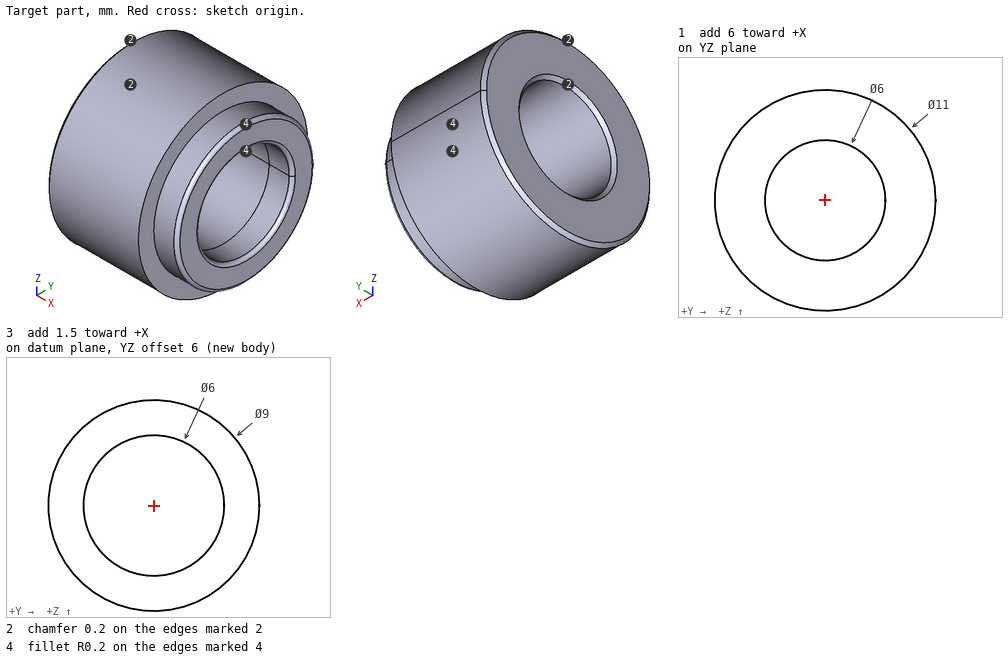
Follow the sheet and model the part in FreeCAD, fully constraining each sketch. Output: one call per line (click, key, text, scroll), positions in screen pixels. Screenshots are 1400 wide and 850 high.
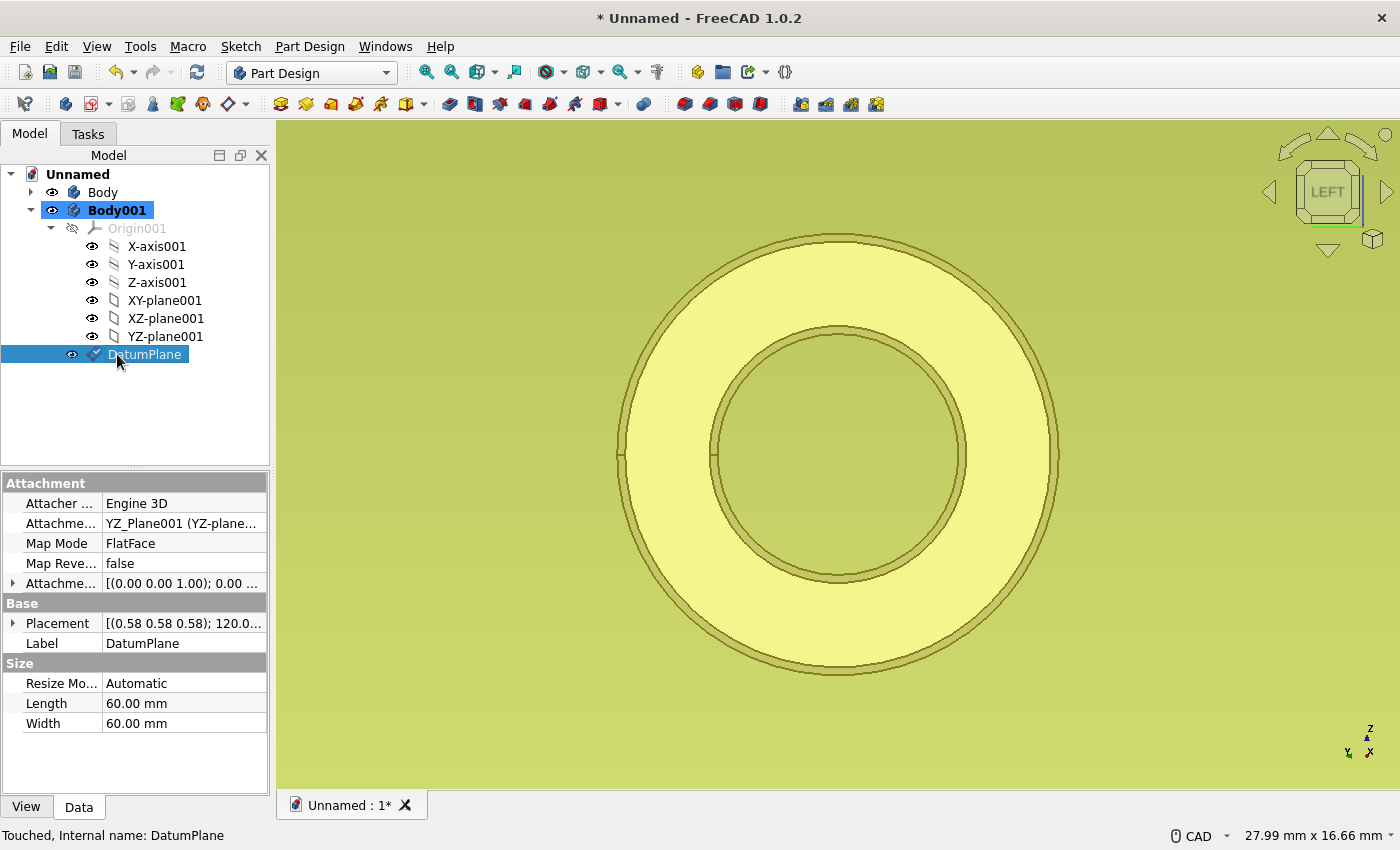
click(90, 104)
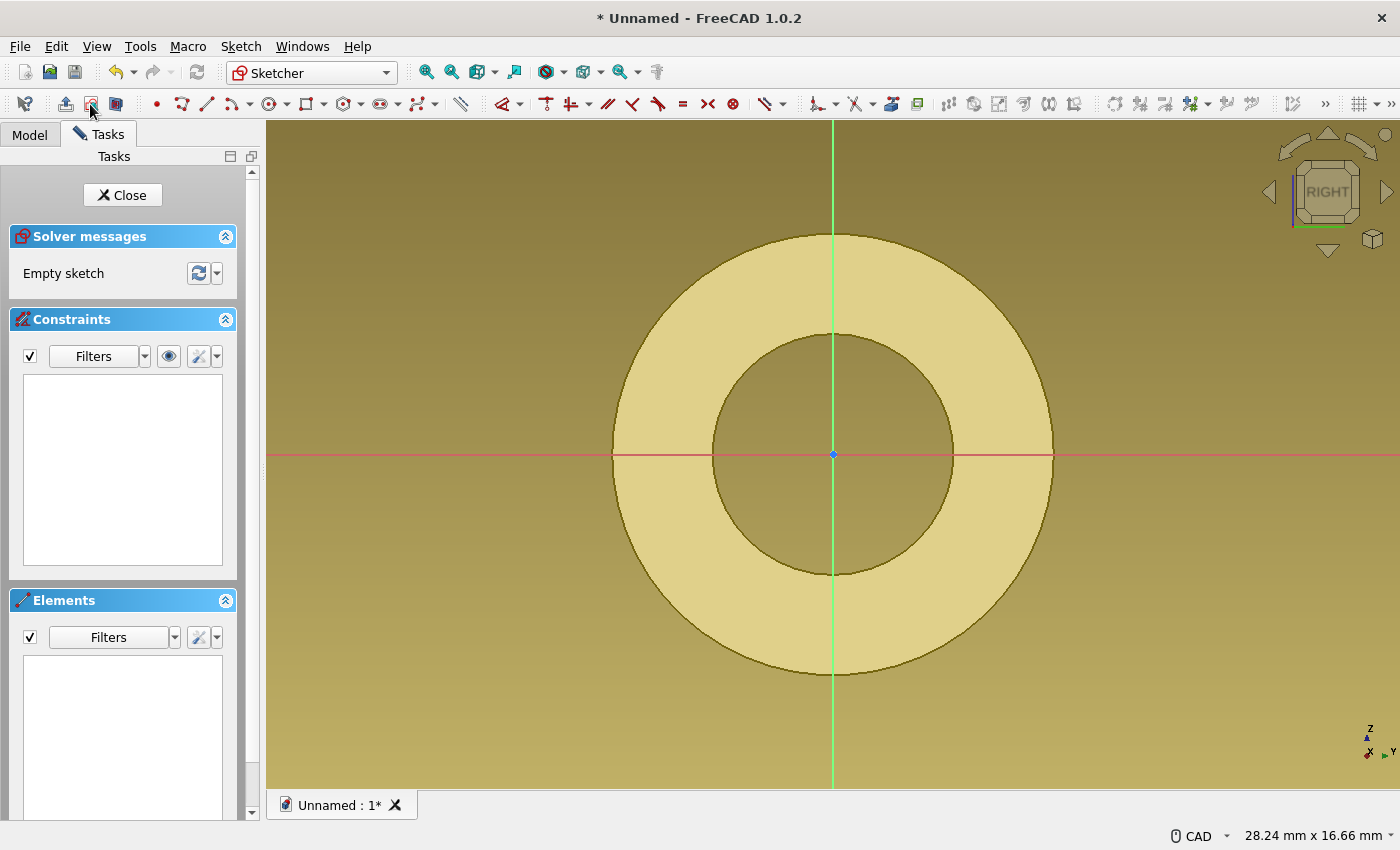
click(268, 104)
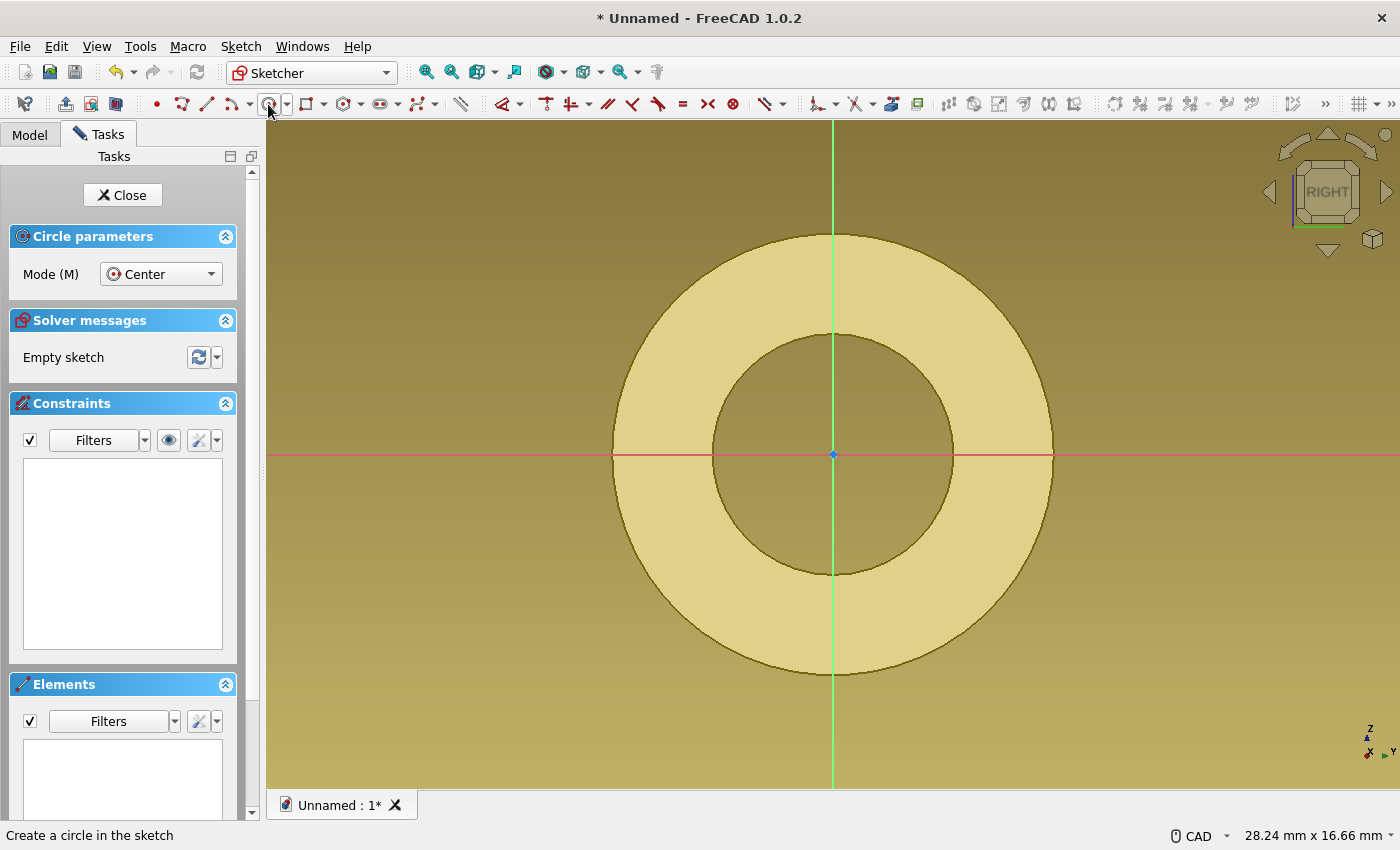
click(833, 454)
move(961, 327)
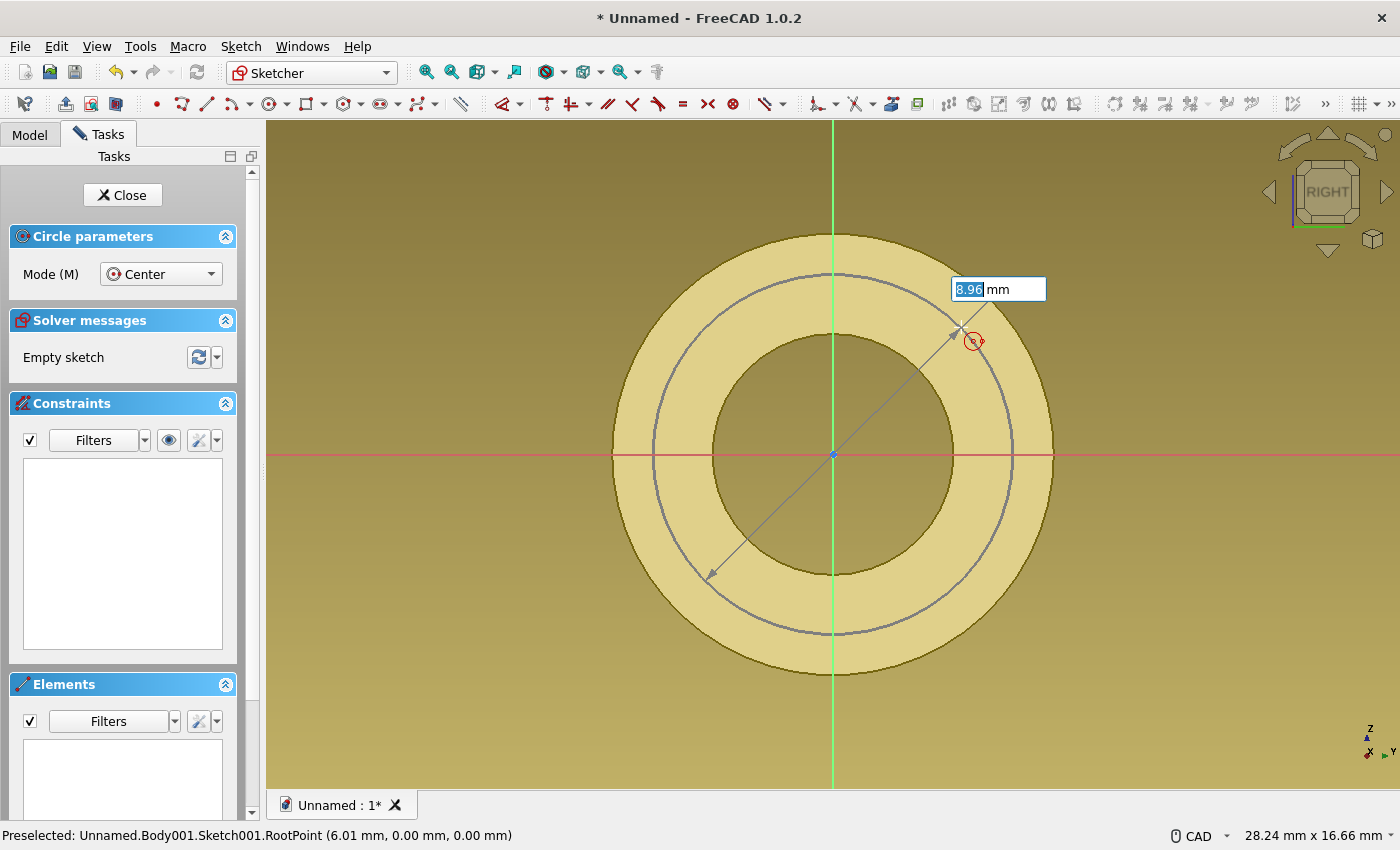
text(9)
key(Return)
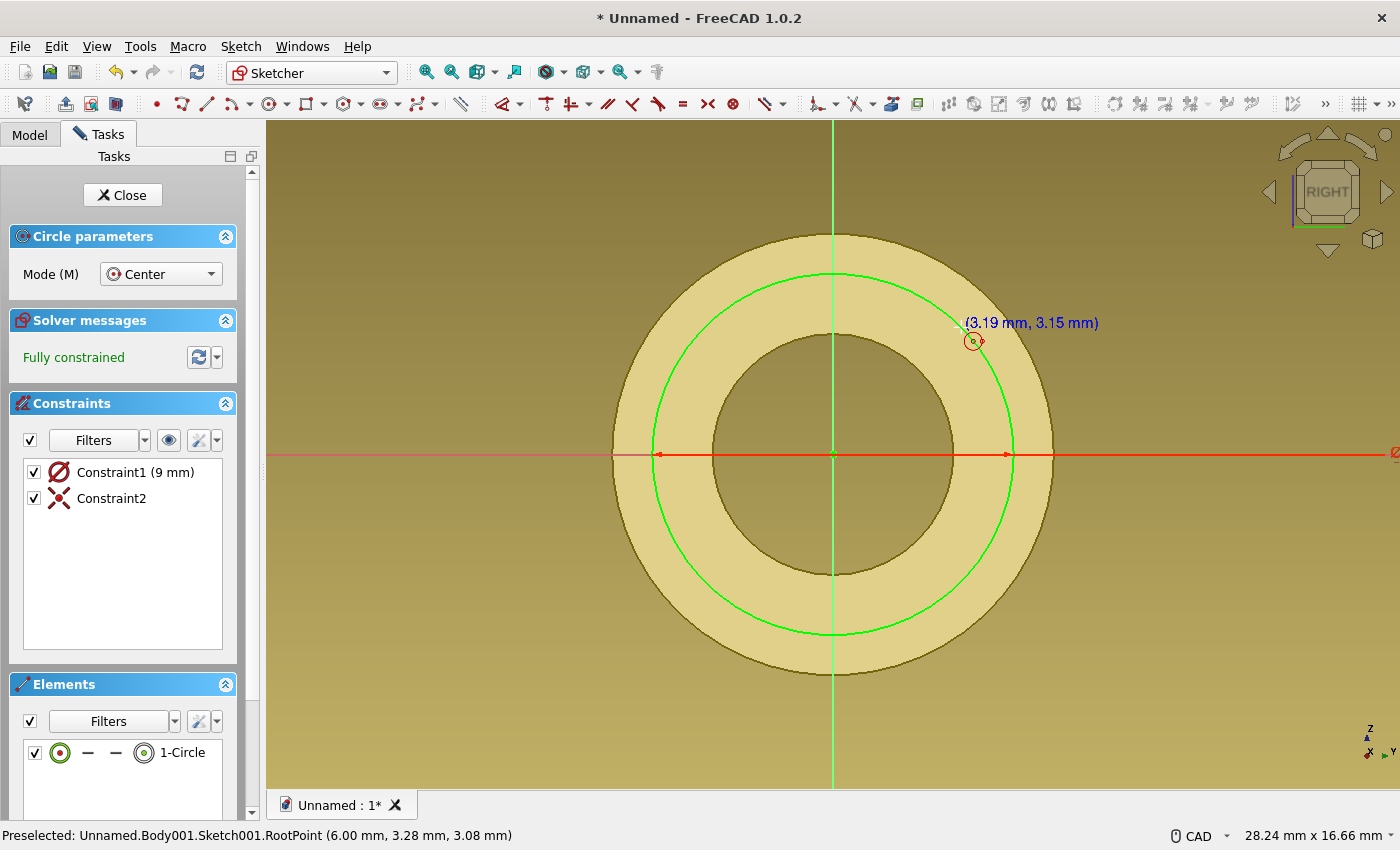
click(833, 454)
move(918, 369)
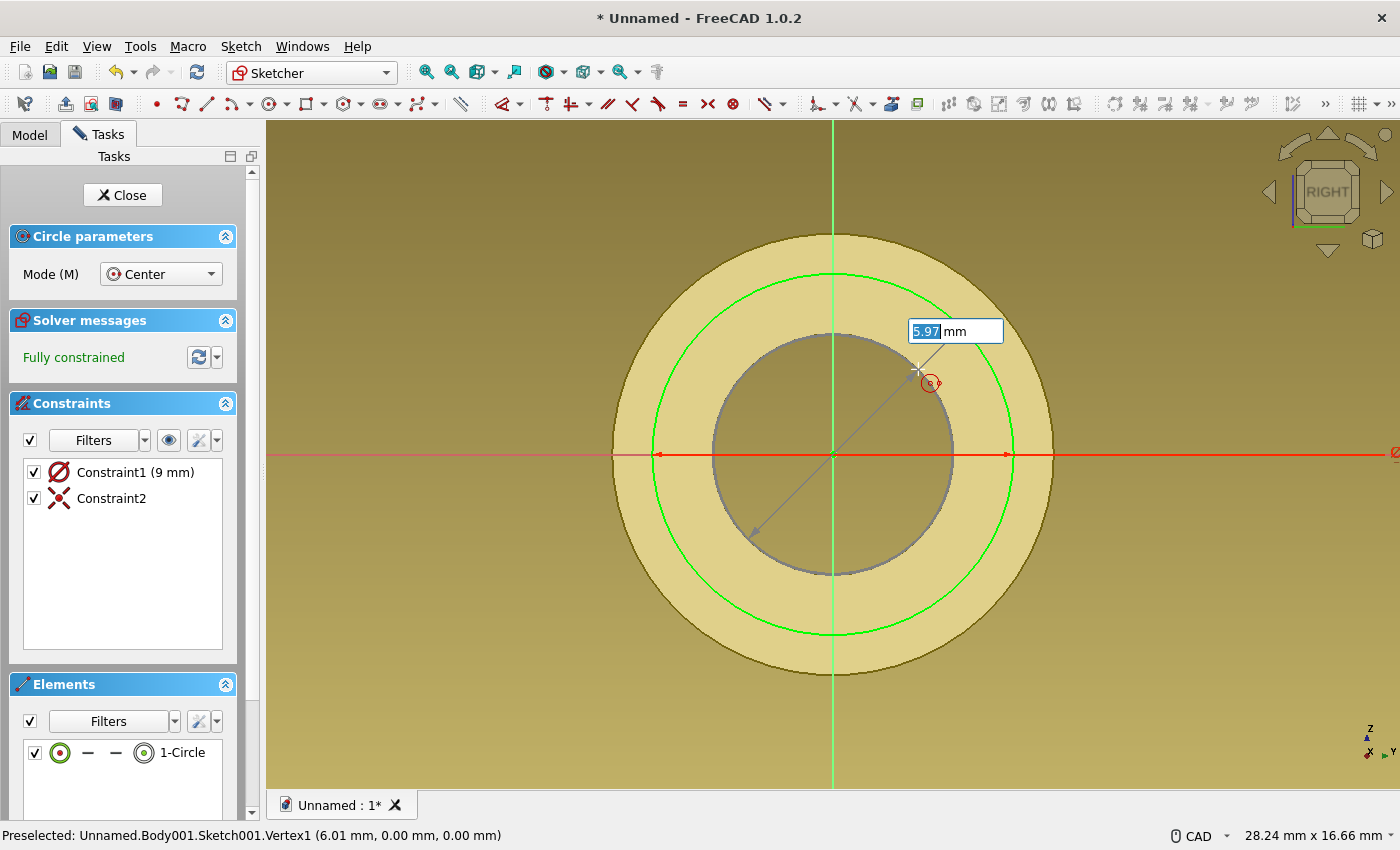
text(6)
key(Return)
key(Escape)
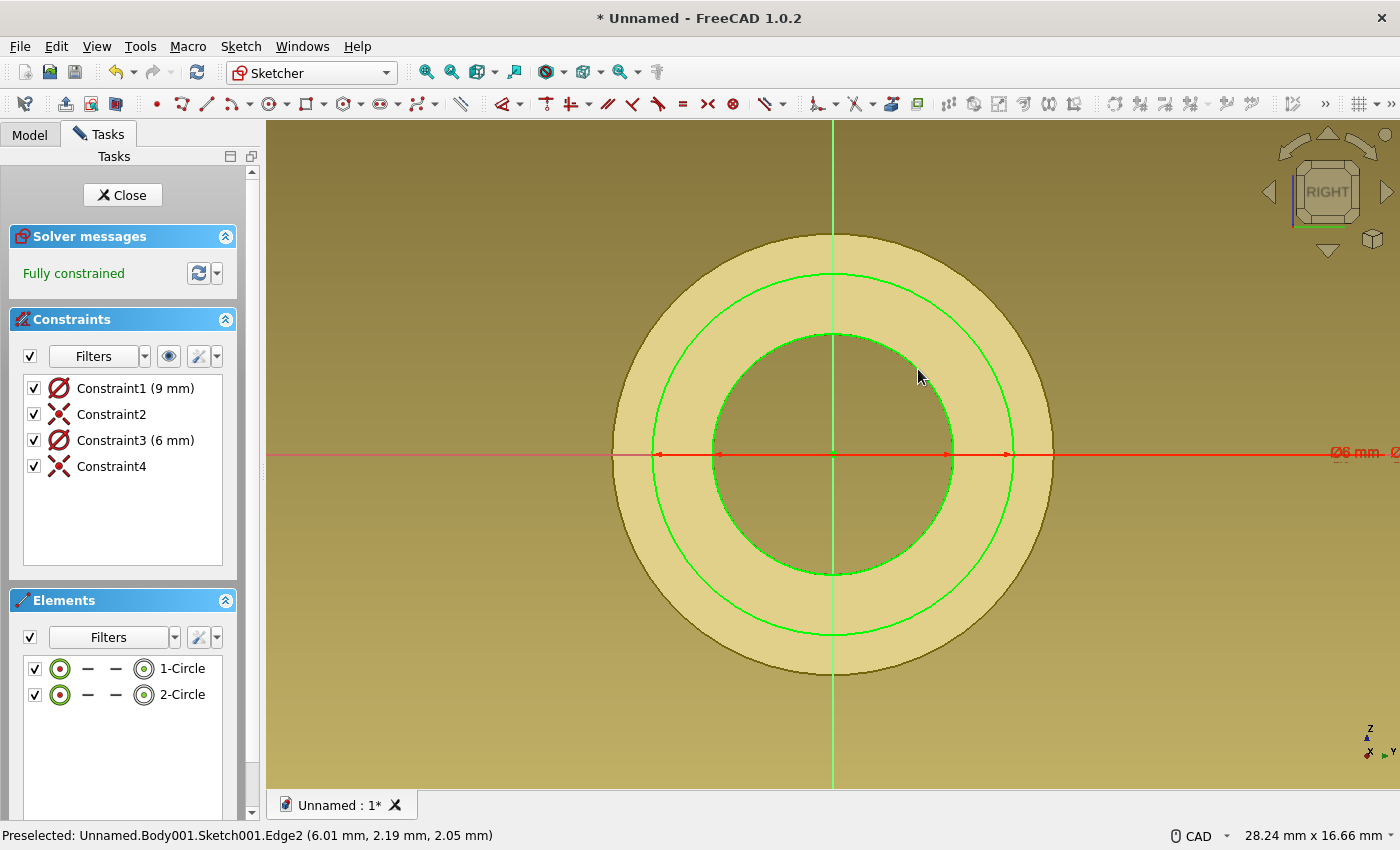
click(123, 195)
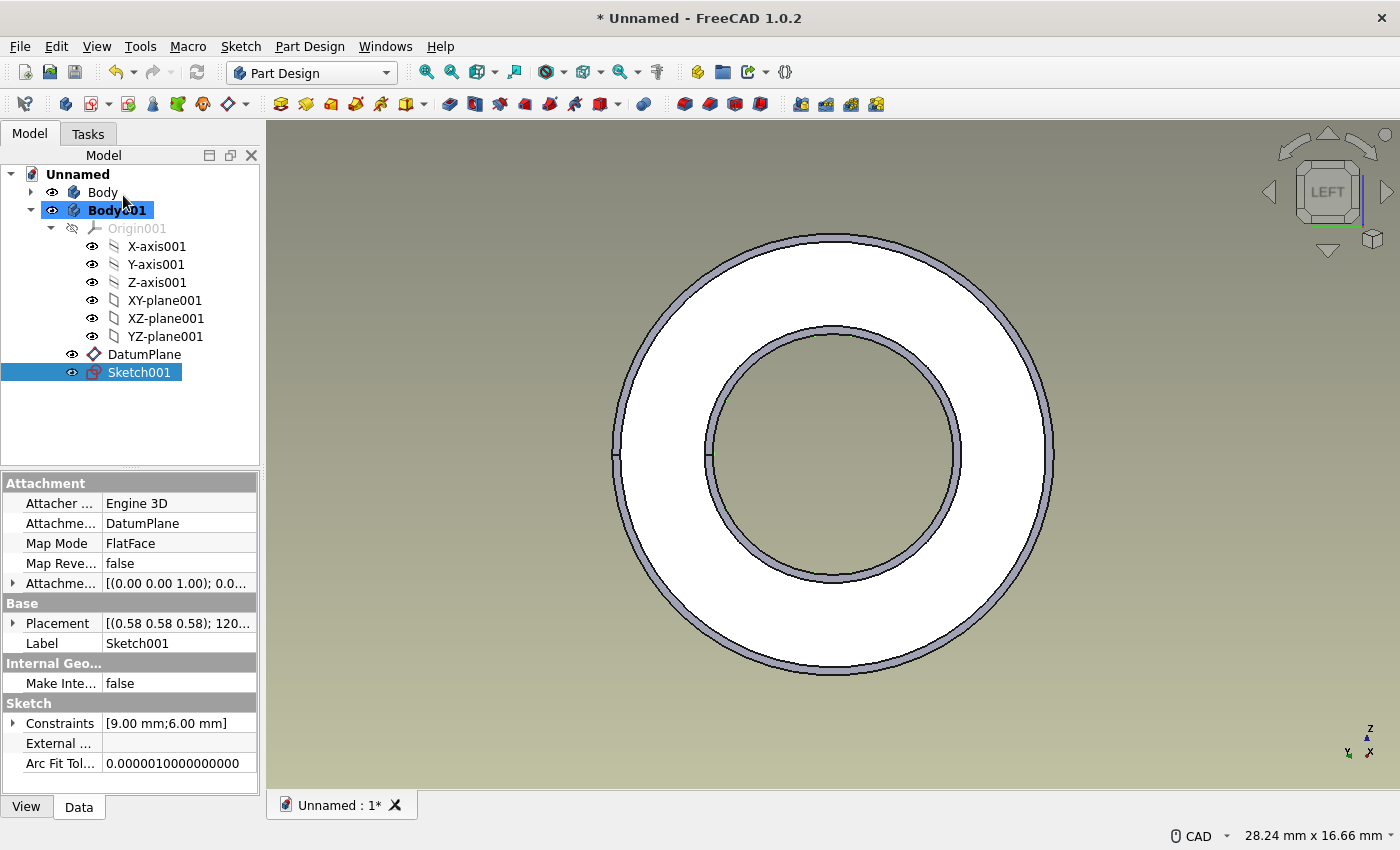
click(281, 104)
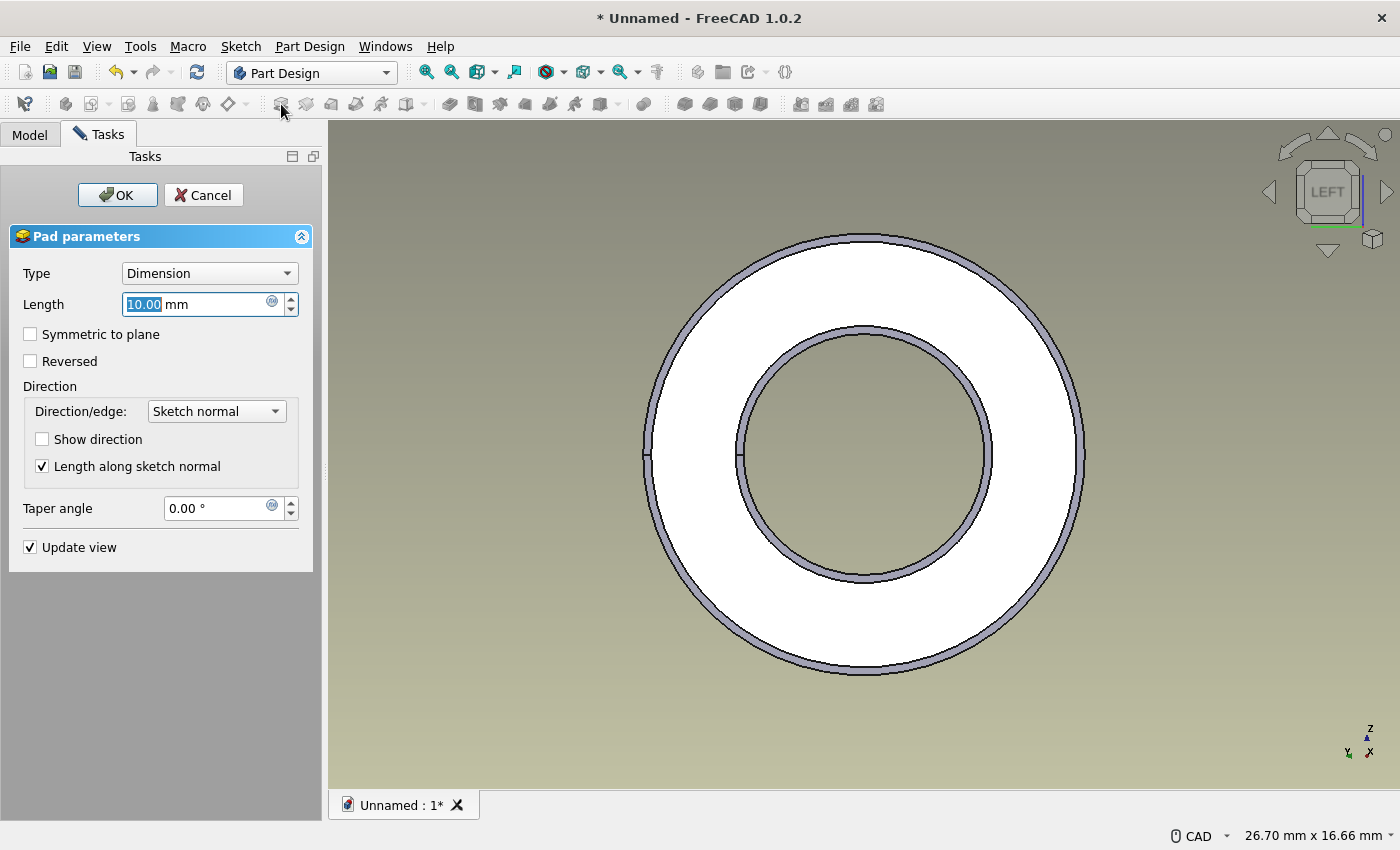
text(1.5)
key(Tab)